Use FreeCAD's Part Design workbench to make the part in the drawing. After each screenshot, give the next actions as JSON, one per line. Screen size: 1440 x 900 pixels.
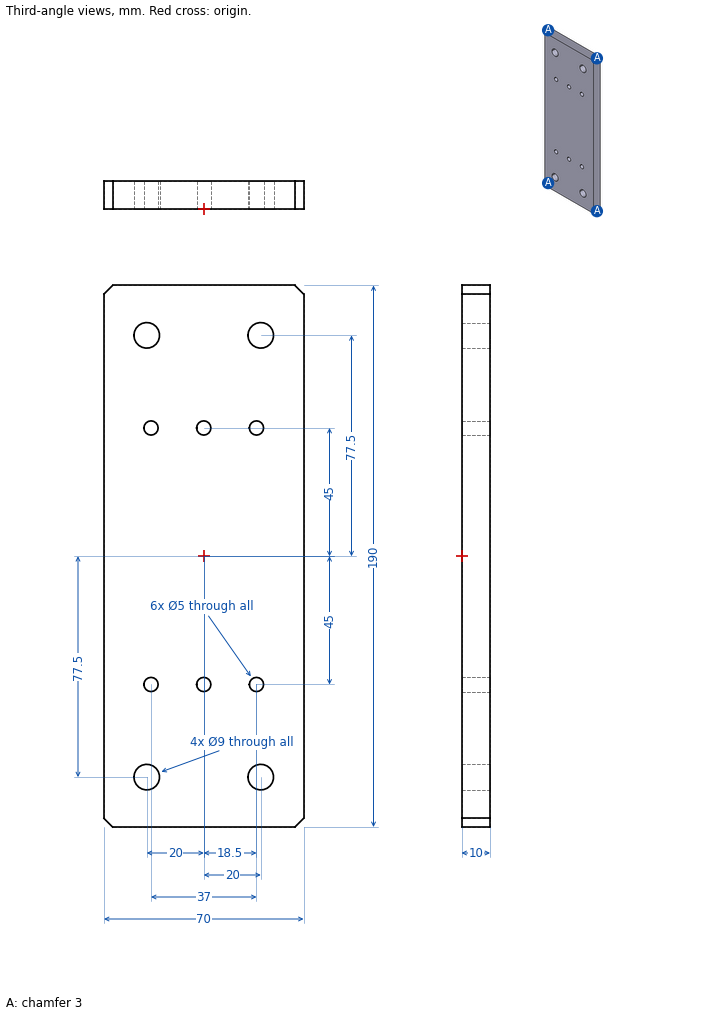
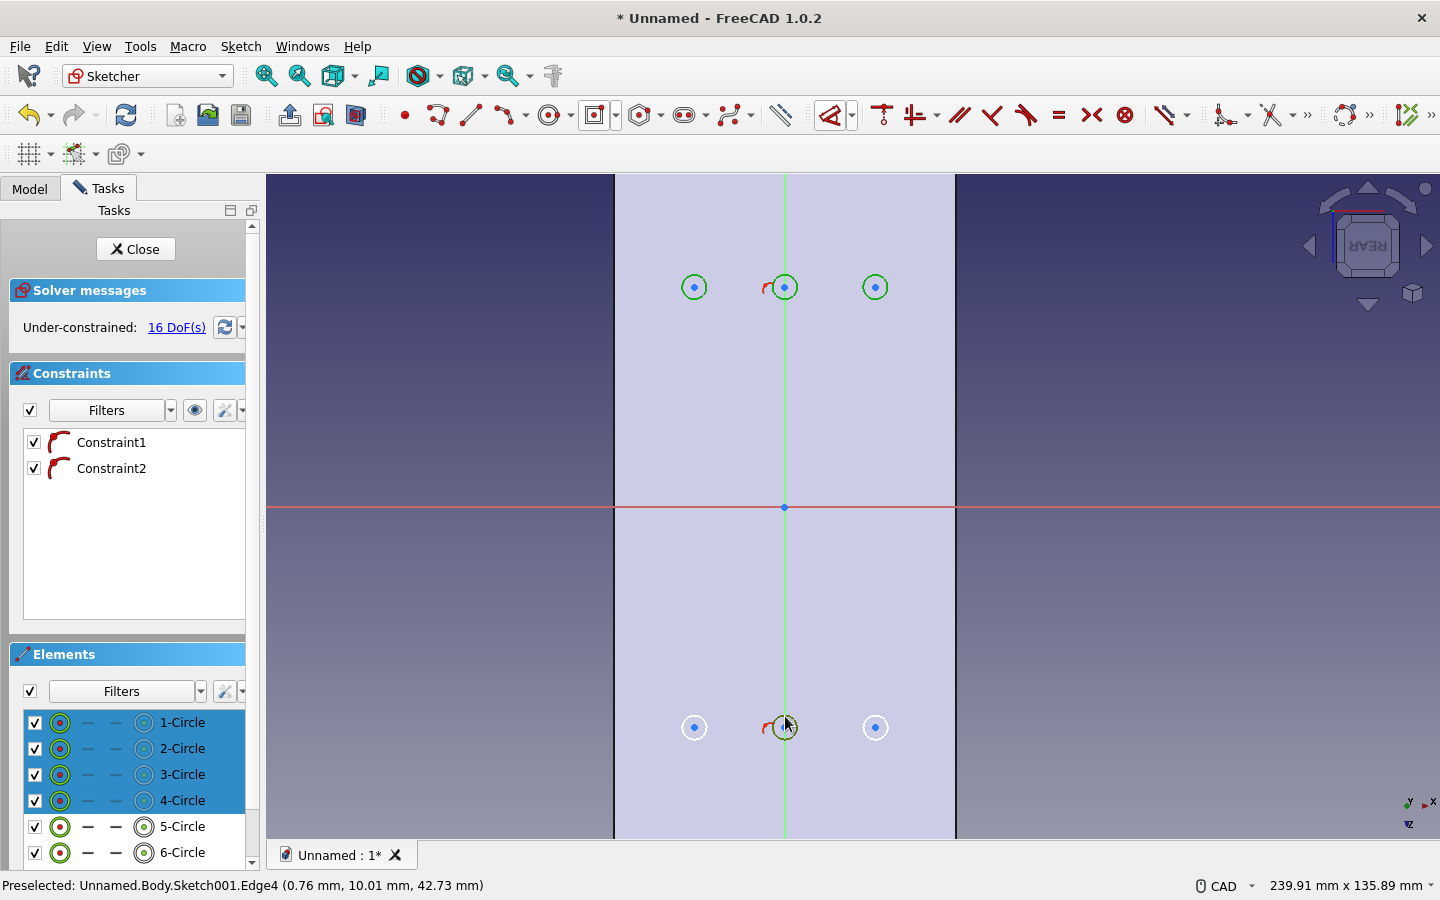
{"action": "left_click", "coordinate": [703, 719]}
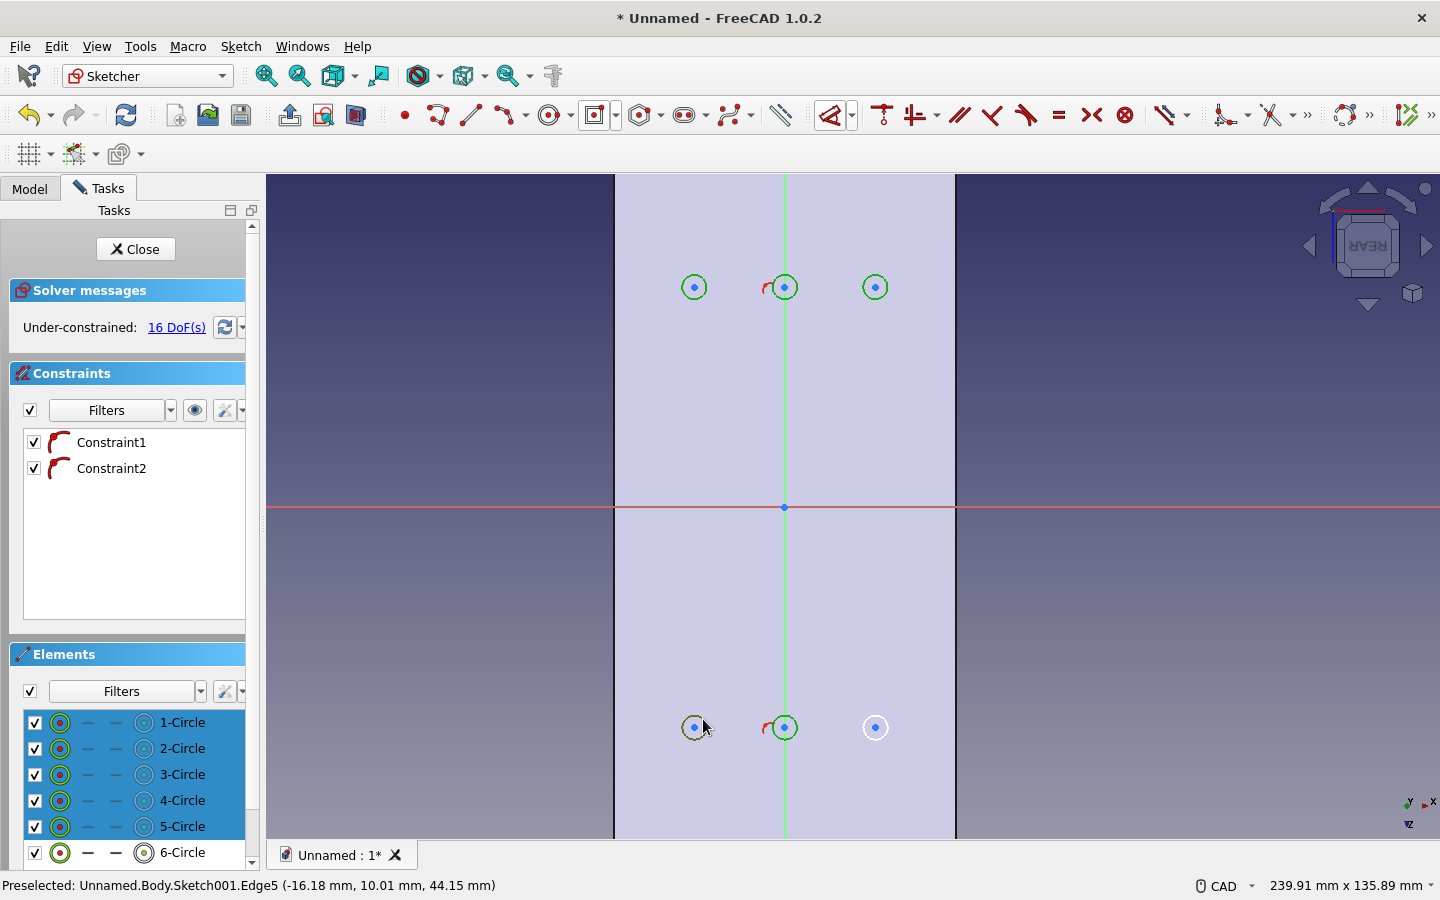
{"action": "left_click", "coordinate": [884, 719]}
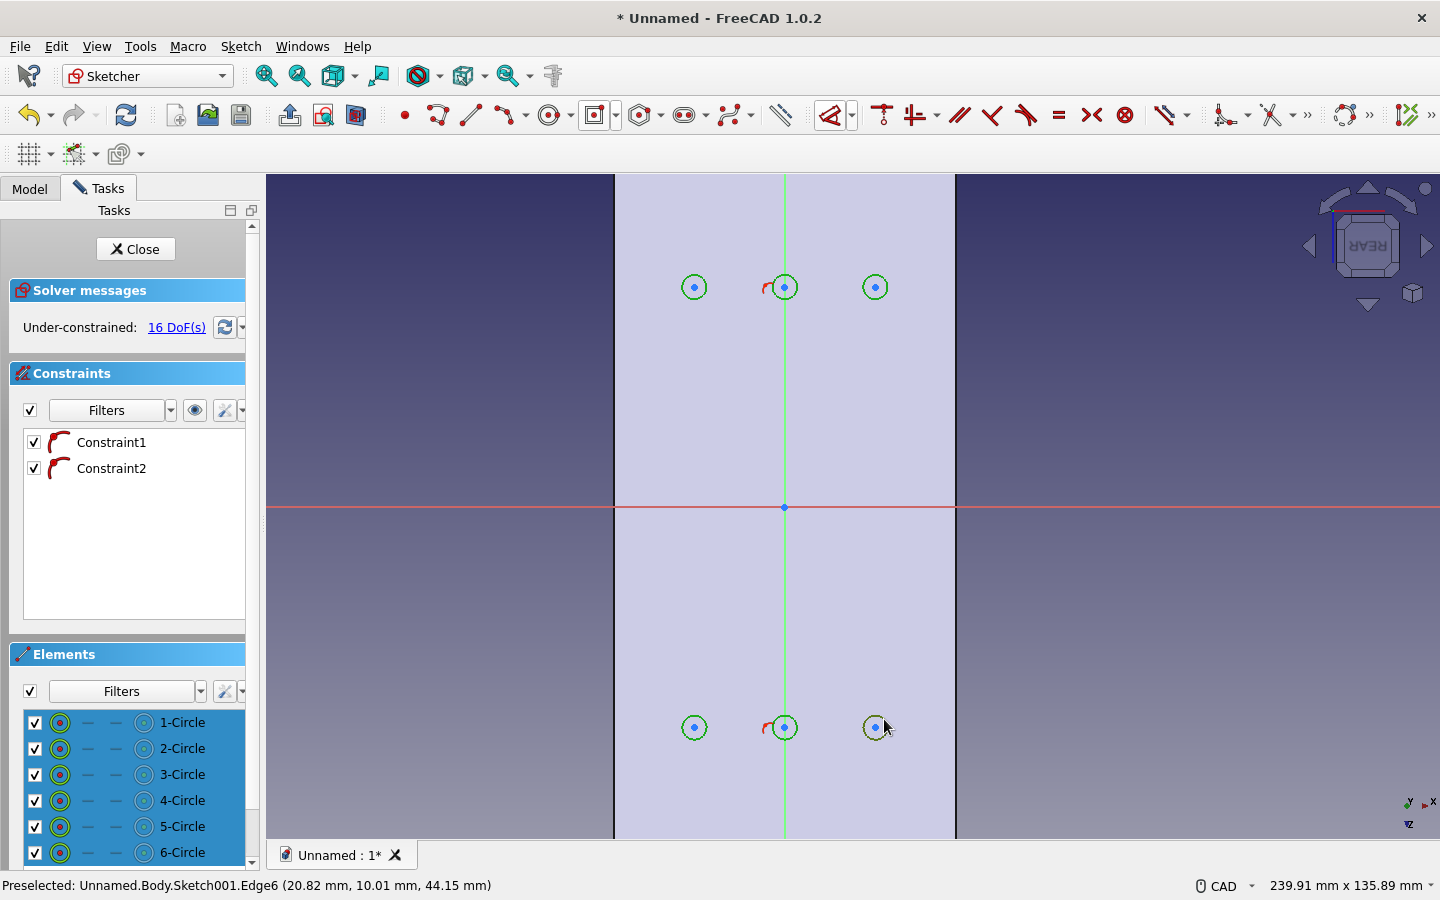
{"action": "left_click", "coordinate": [1059, 116]}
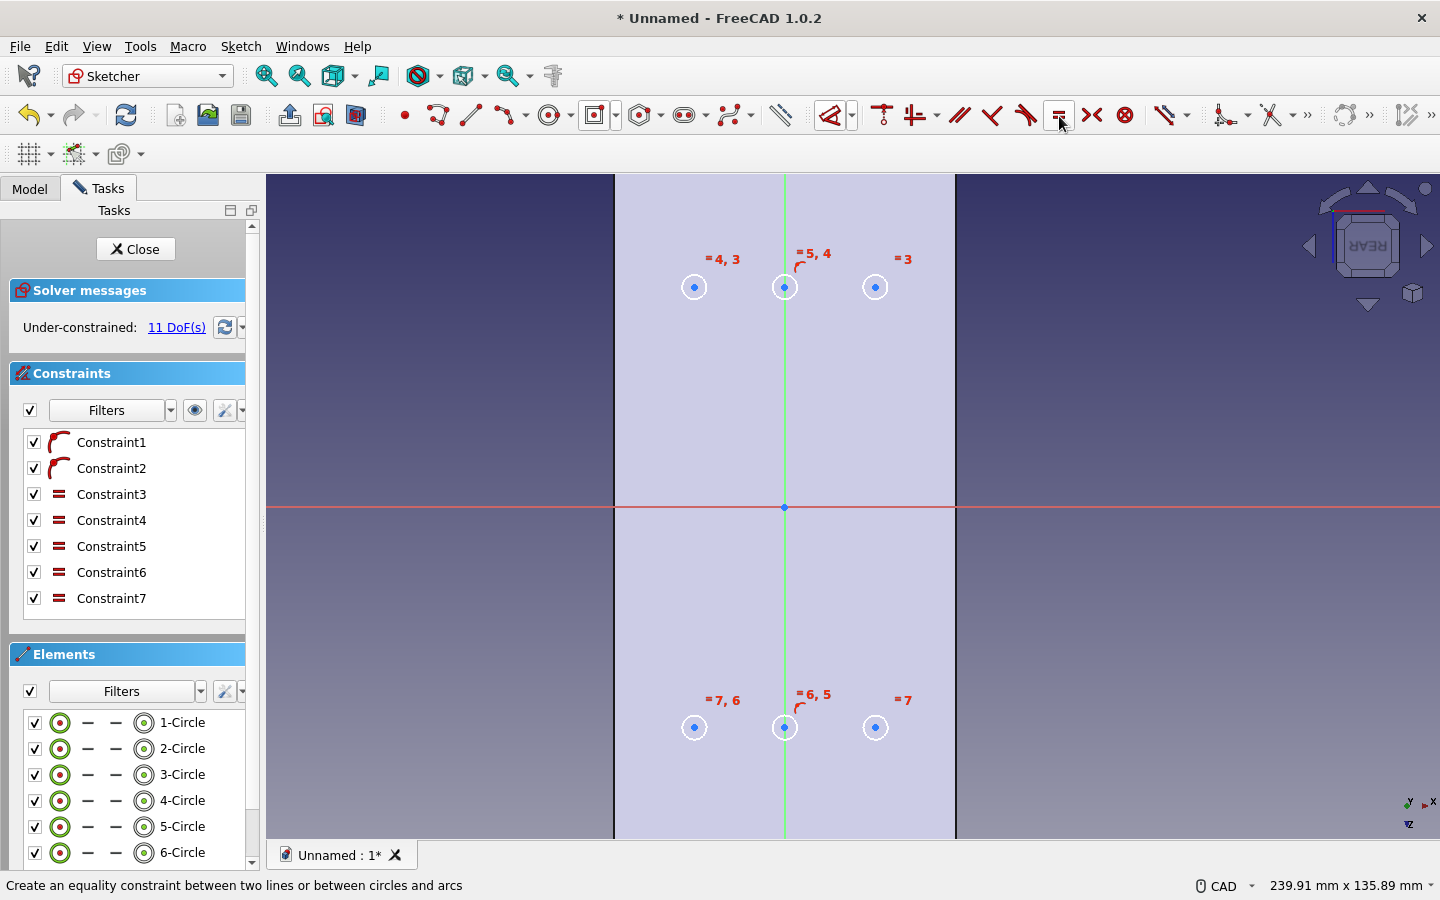
{"action": "left_click", "coordinate": [875, 287]}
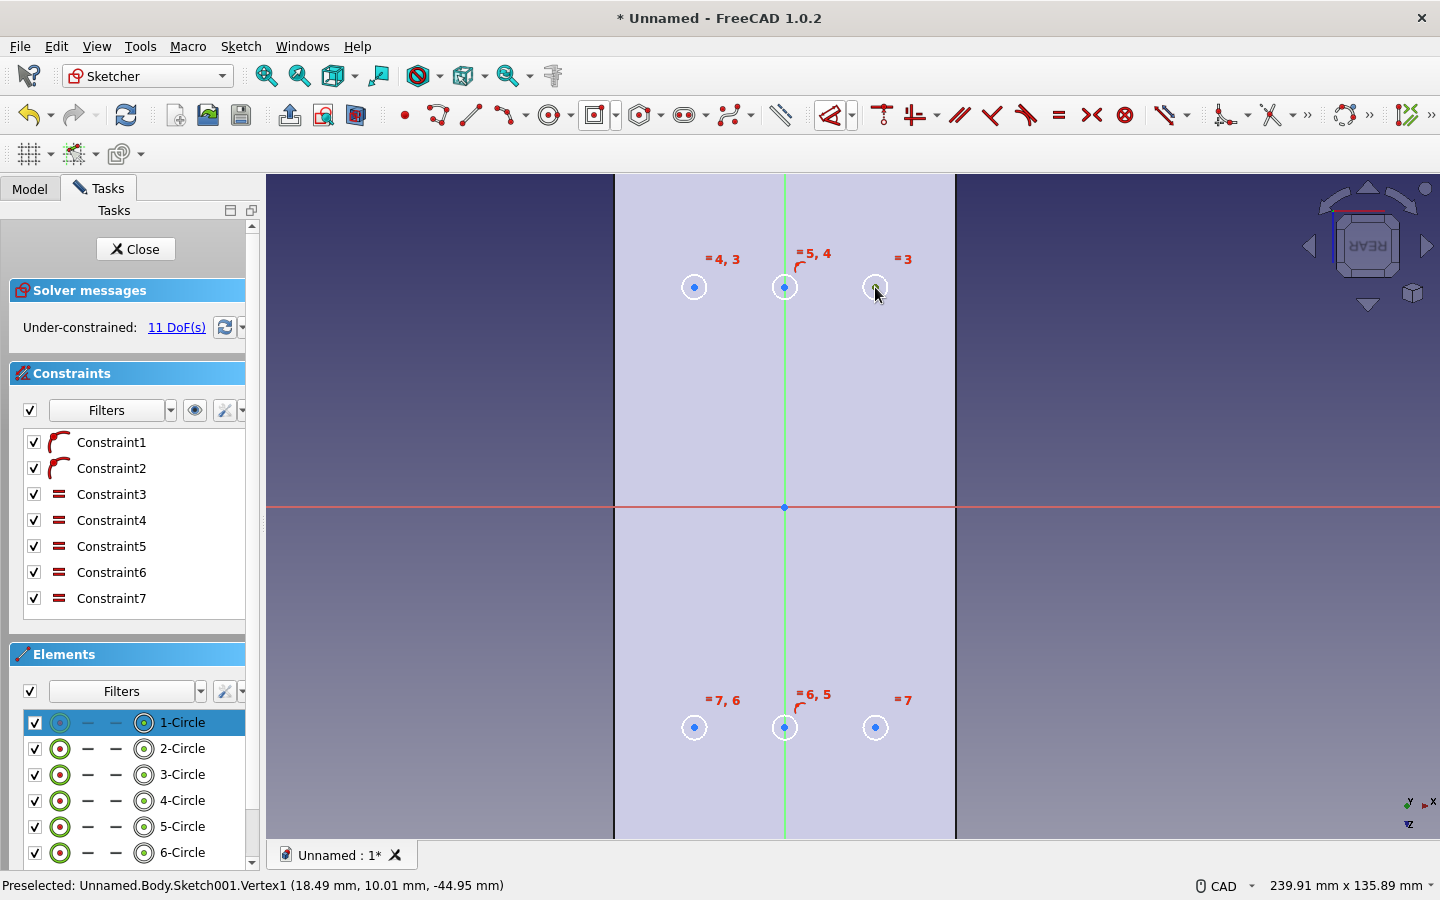
{"action": "left_click", "coordinate": [694, 287]}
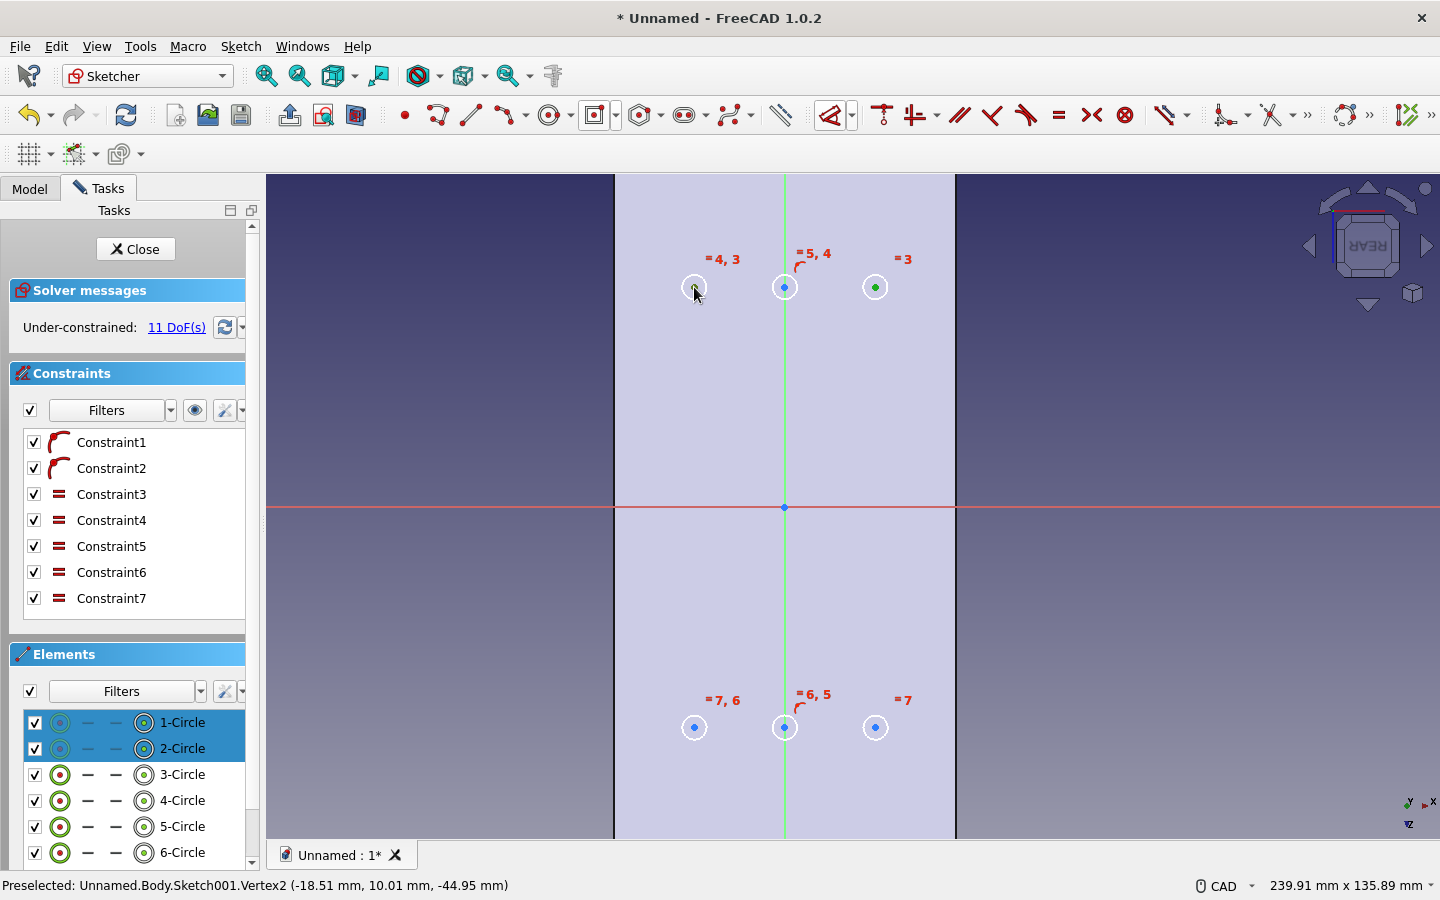
{"action": "key", "text": "h"}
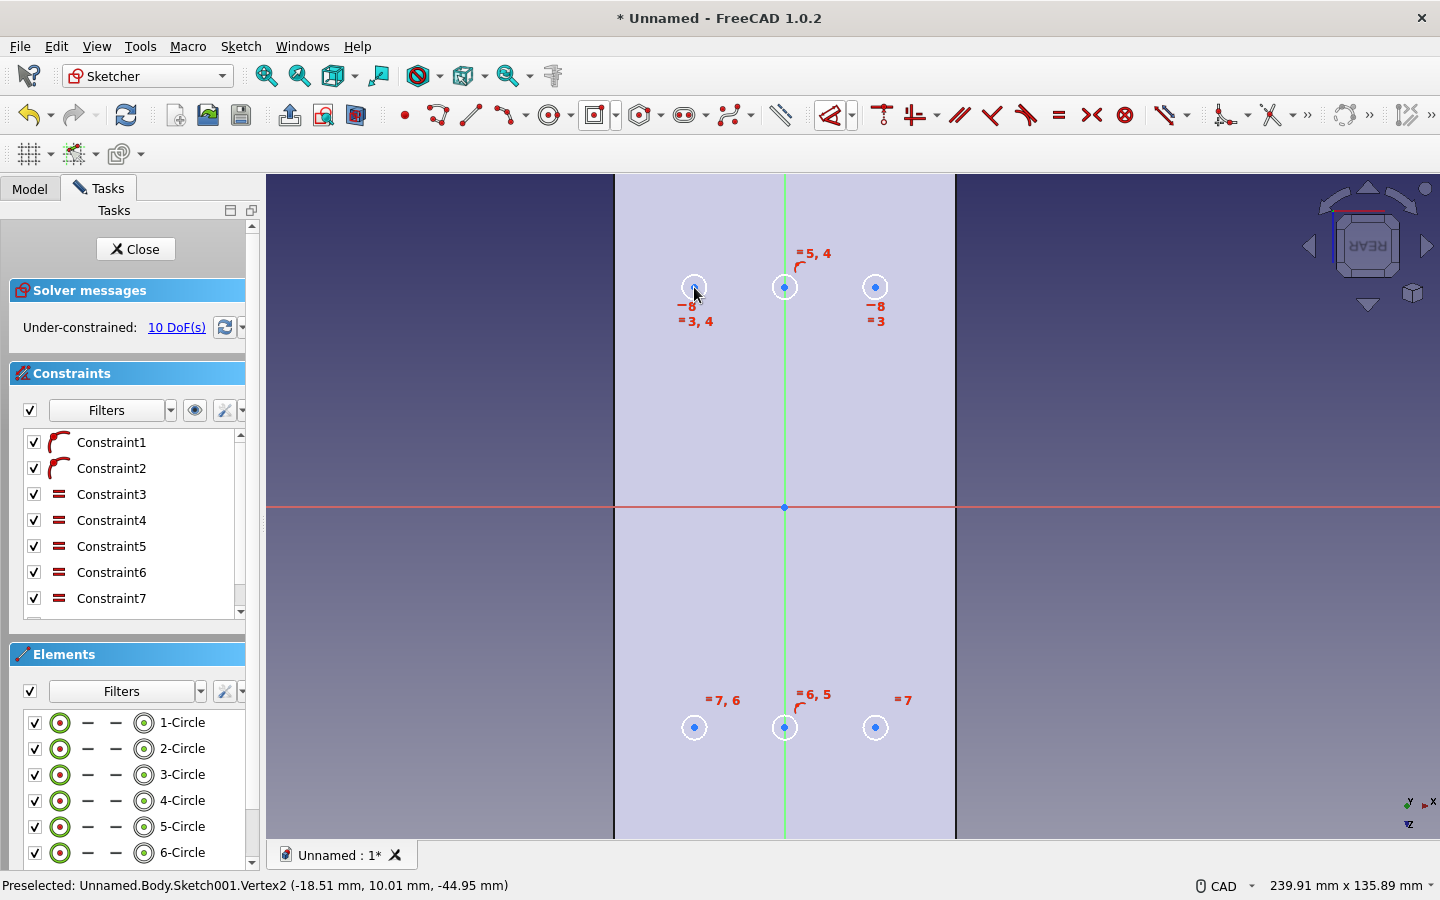
{"action": "left_click", "coordinate": [875, 287]}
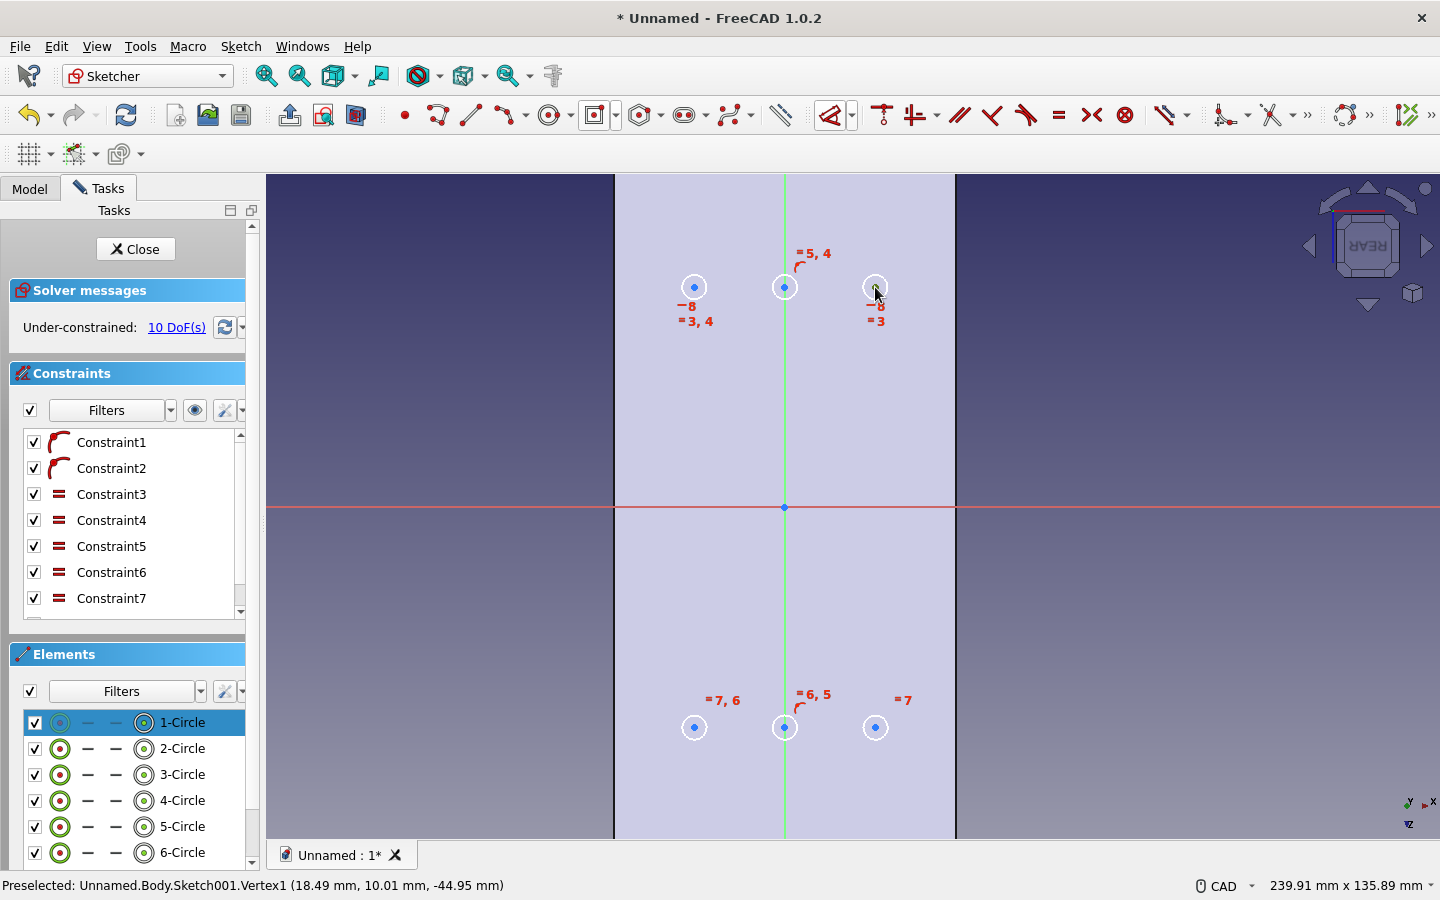
{"action": "left_click", "coordinate": [785, 287]}